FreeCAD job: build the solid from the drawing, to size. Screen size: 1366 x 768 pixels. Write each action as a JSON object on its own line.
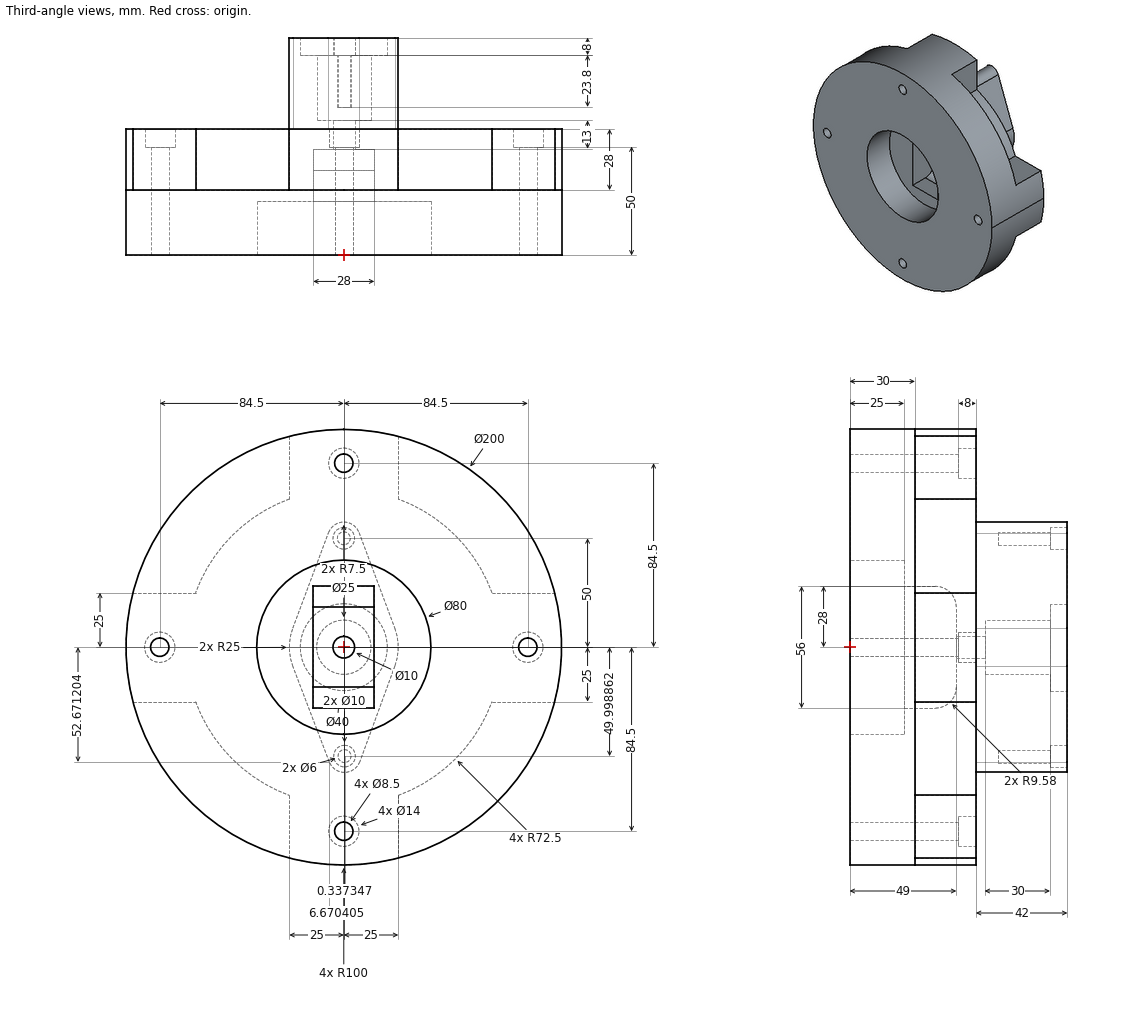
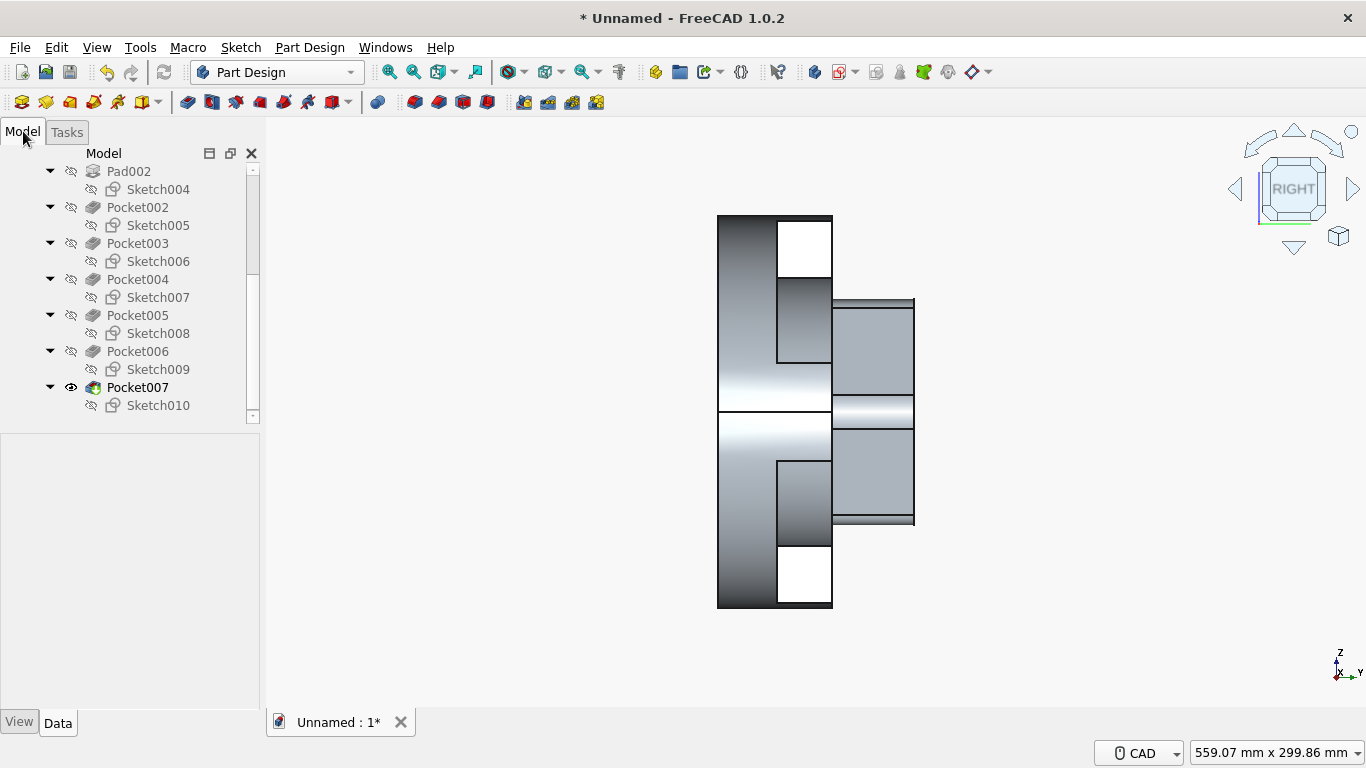
{"action": "scroll", "coordinate": [140, 293], "scroll_direction": "down", "scroll_amount": 3}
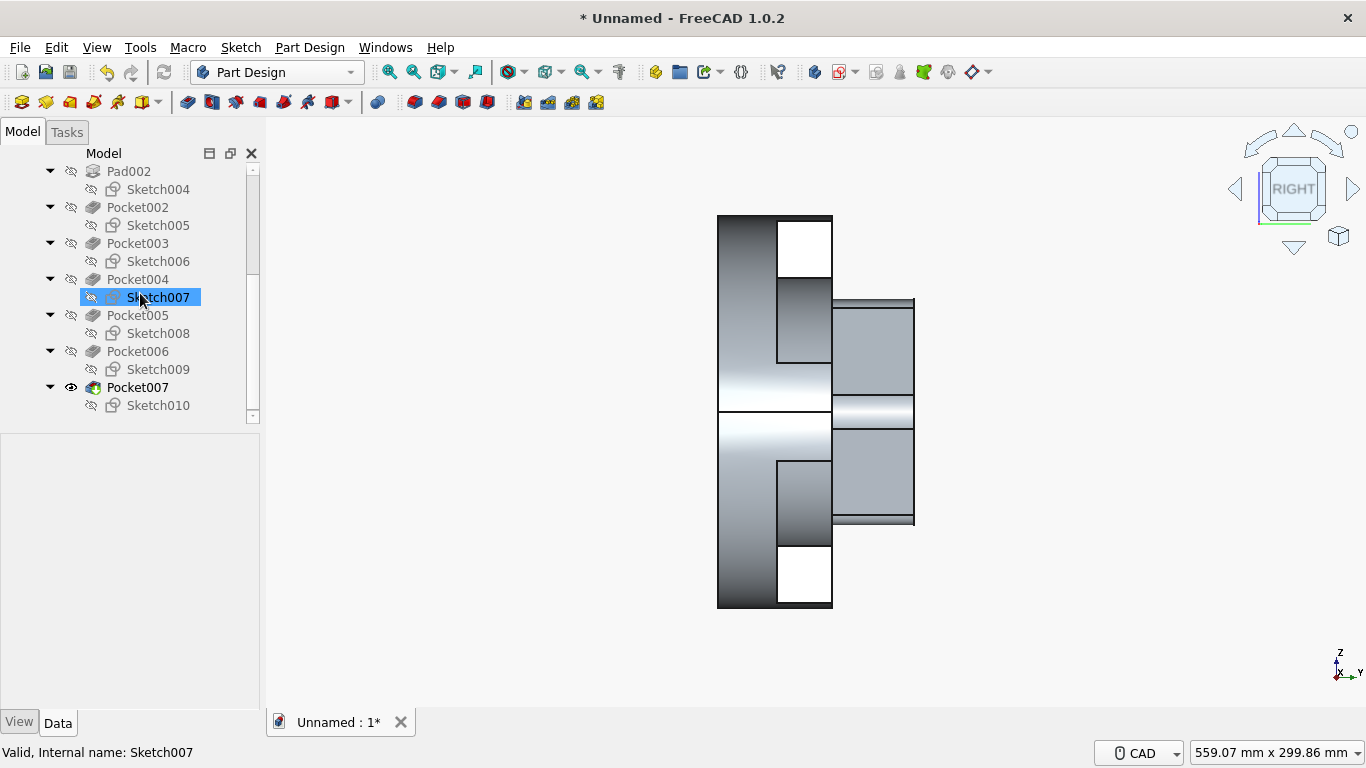
{"action": "scroll", "coordinate": [140, 293], "scroll_direction": "up", "scroll_amount": 15}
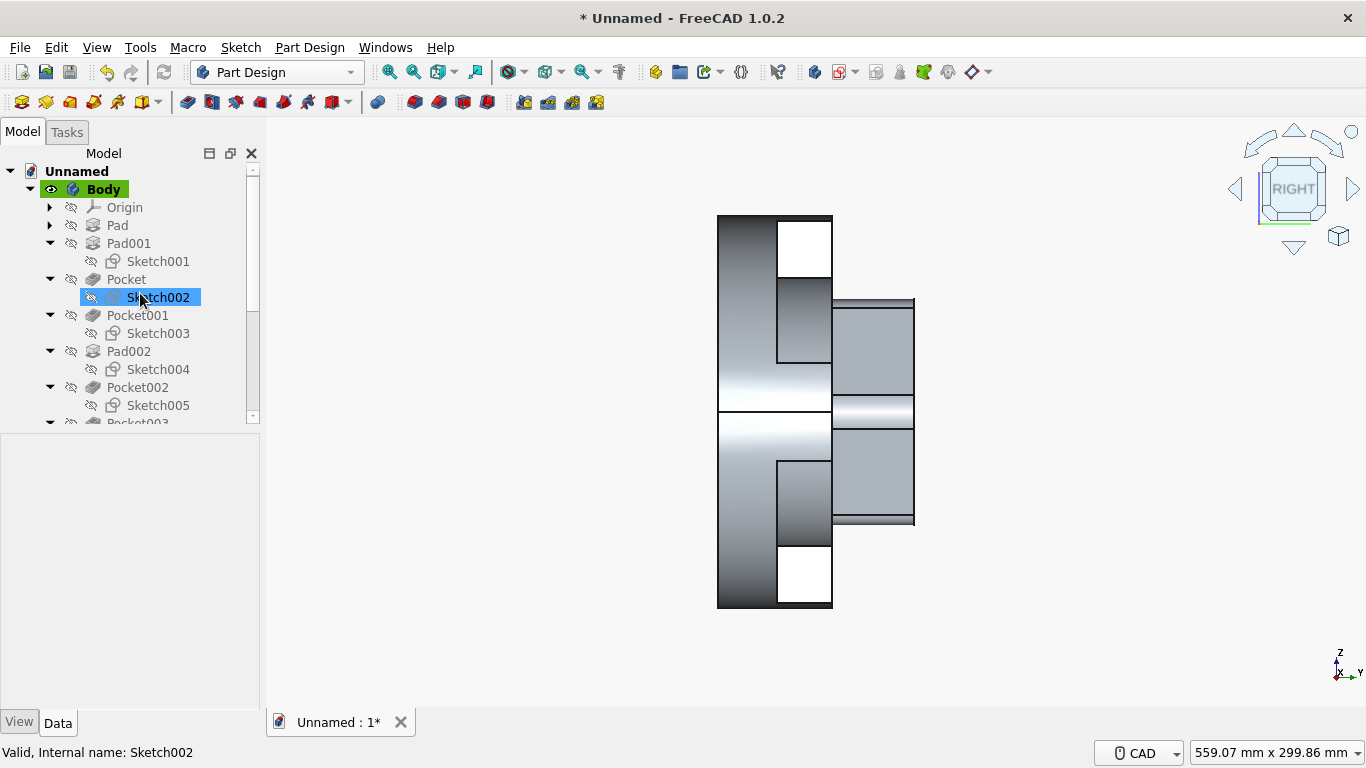
{"action": "left_click", "coordinate": [50, 207]}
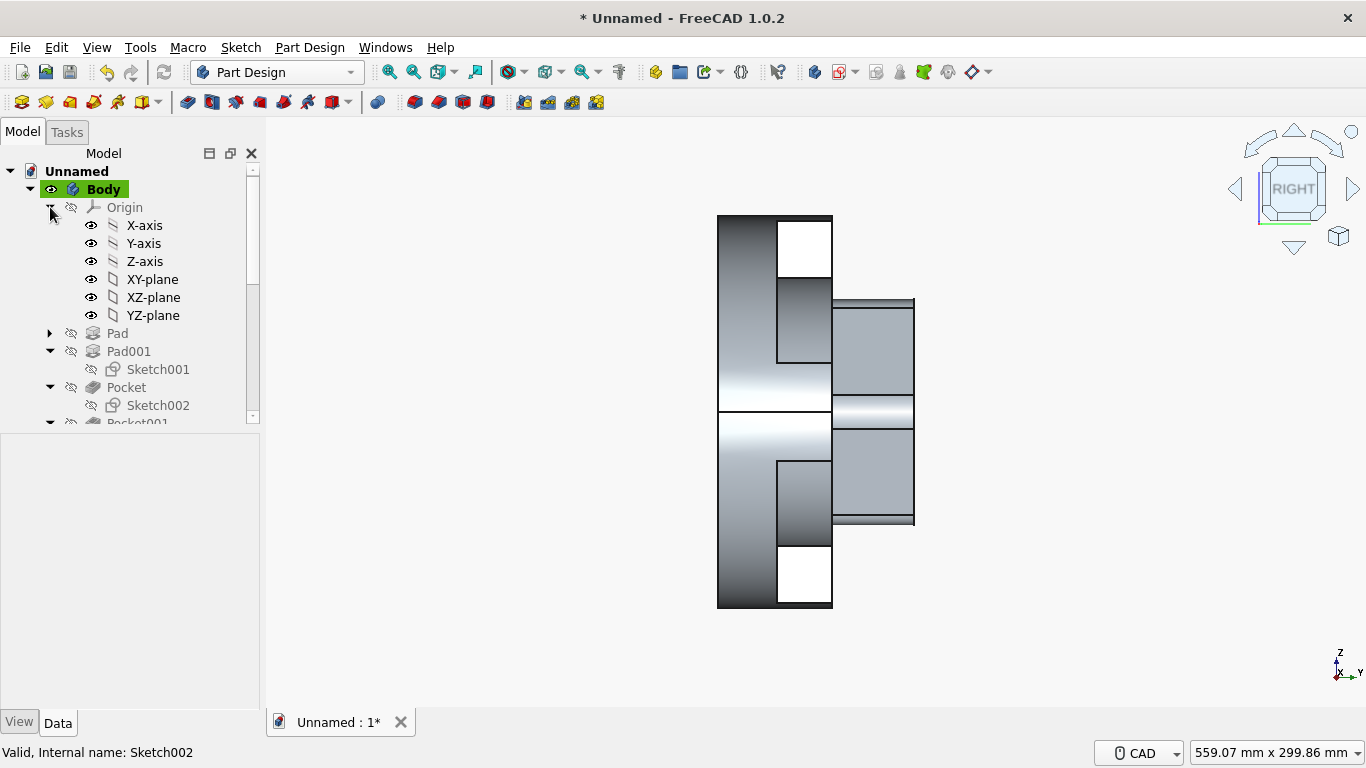
{"action": "left_click", "coordinate": [136, 297]}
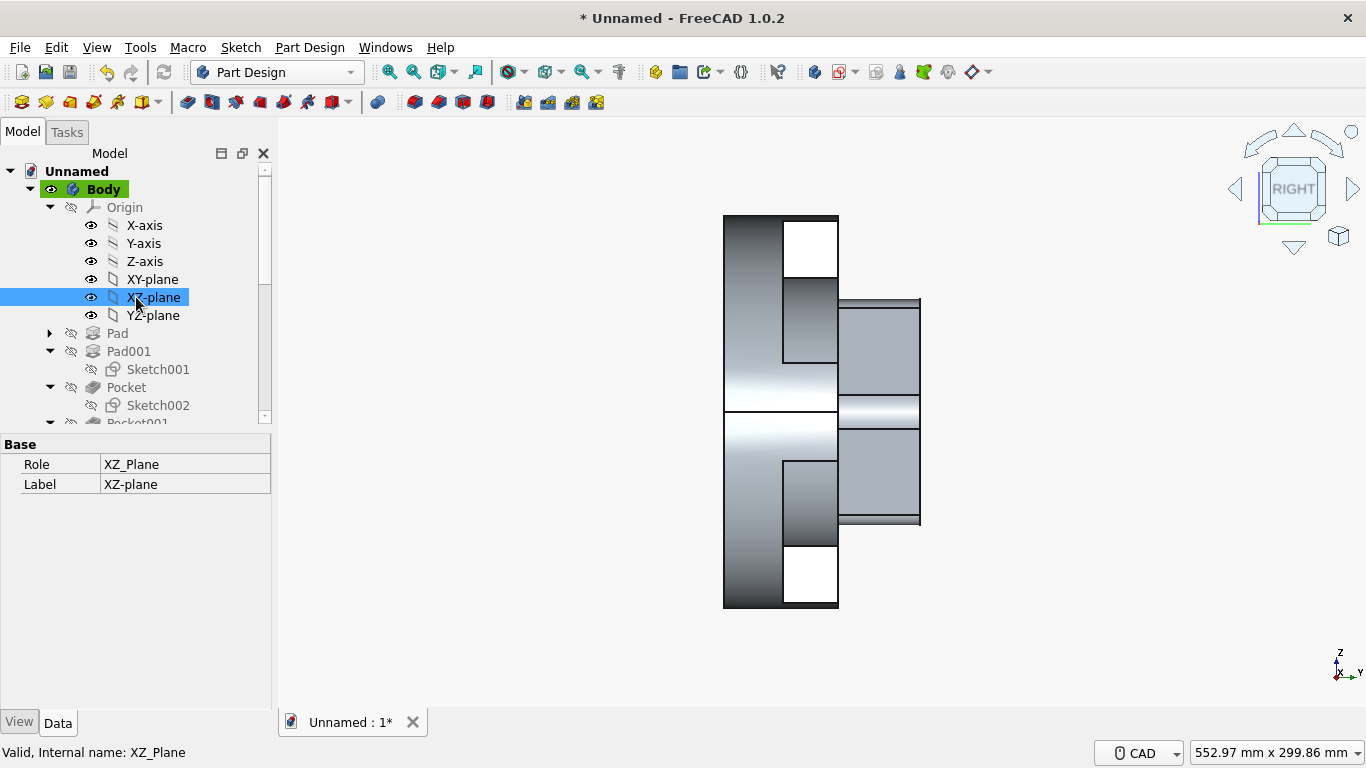
{"action": "left_click", "coordinate": [972, 72]}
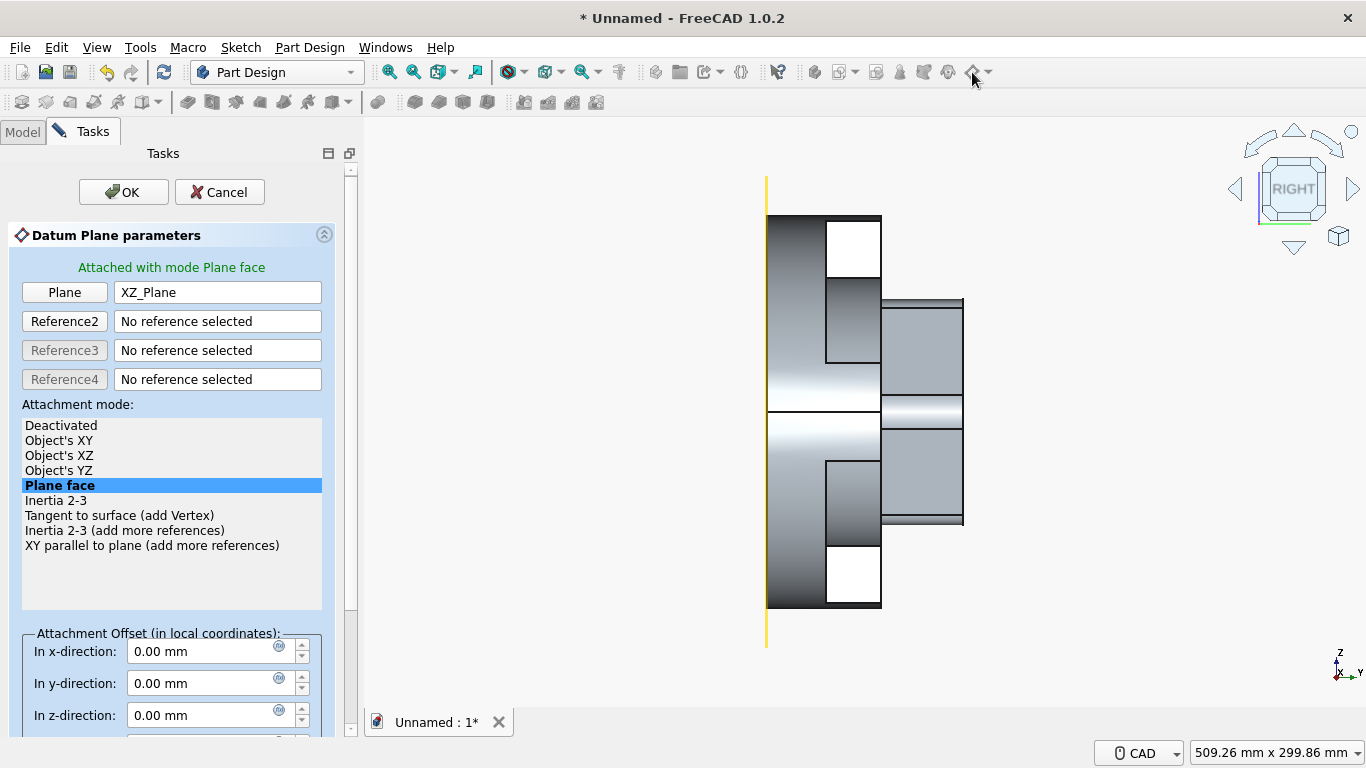
{"action": "triple_click", "coordinate": [210, 715]}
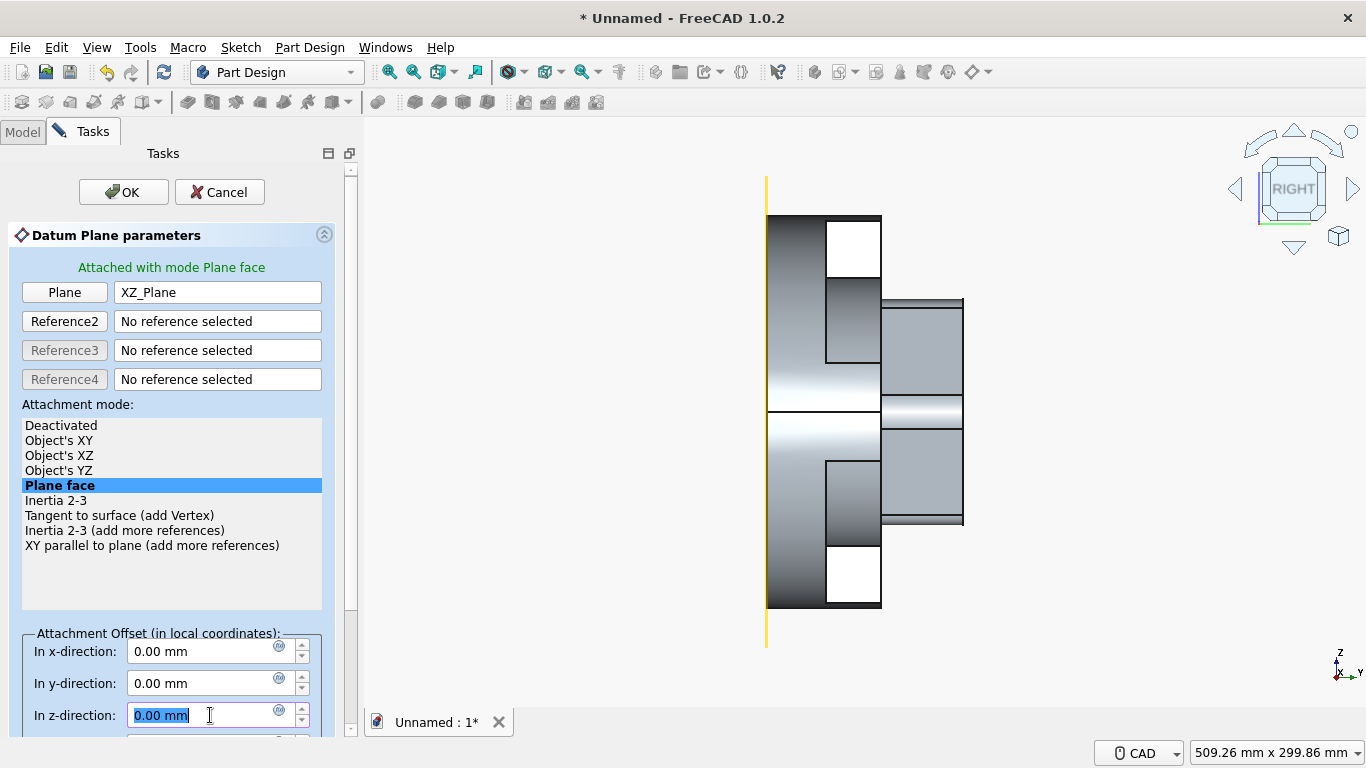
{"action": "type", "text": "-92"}
{"action": "key", "text": "Tab"}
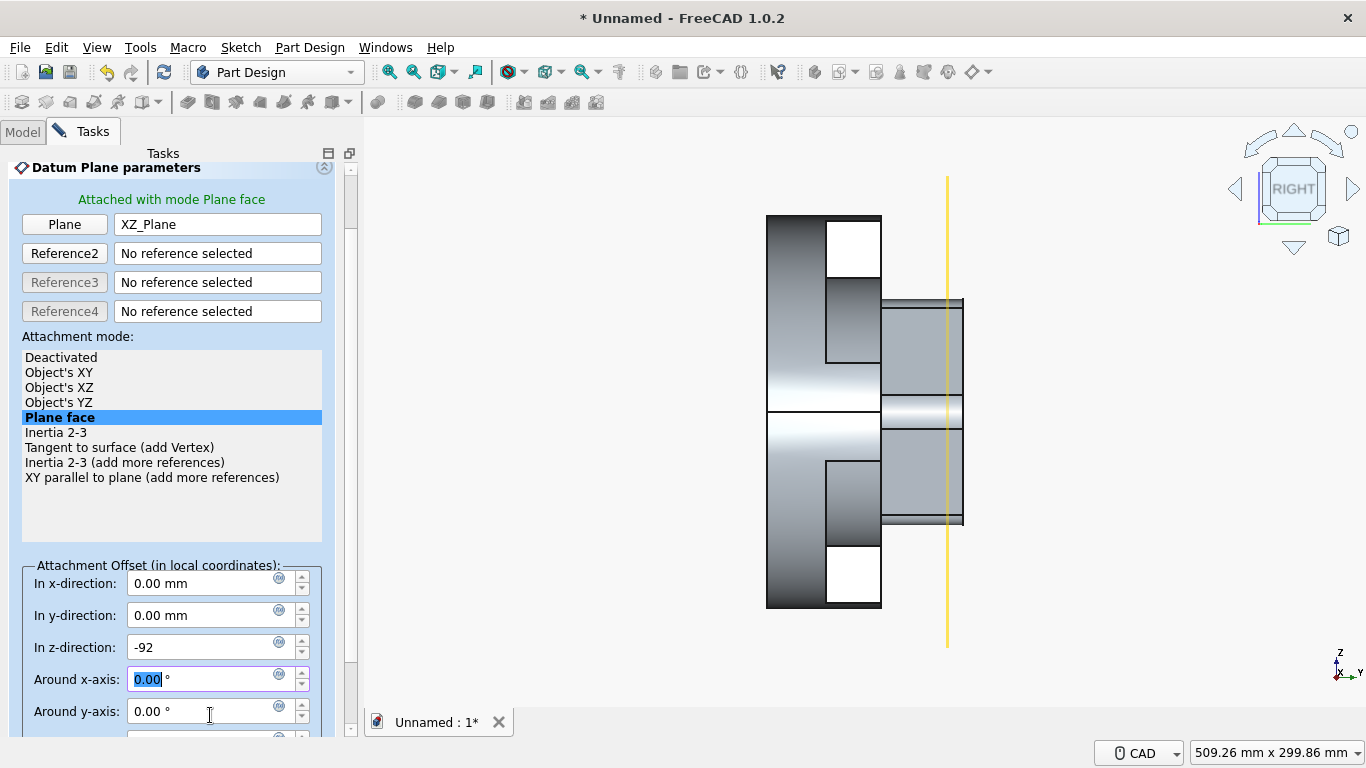
{"action": "scroll", "coordinate": [351, 450], "scroll_direction": "up", "scroll_amount": 2}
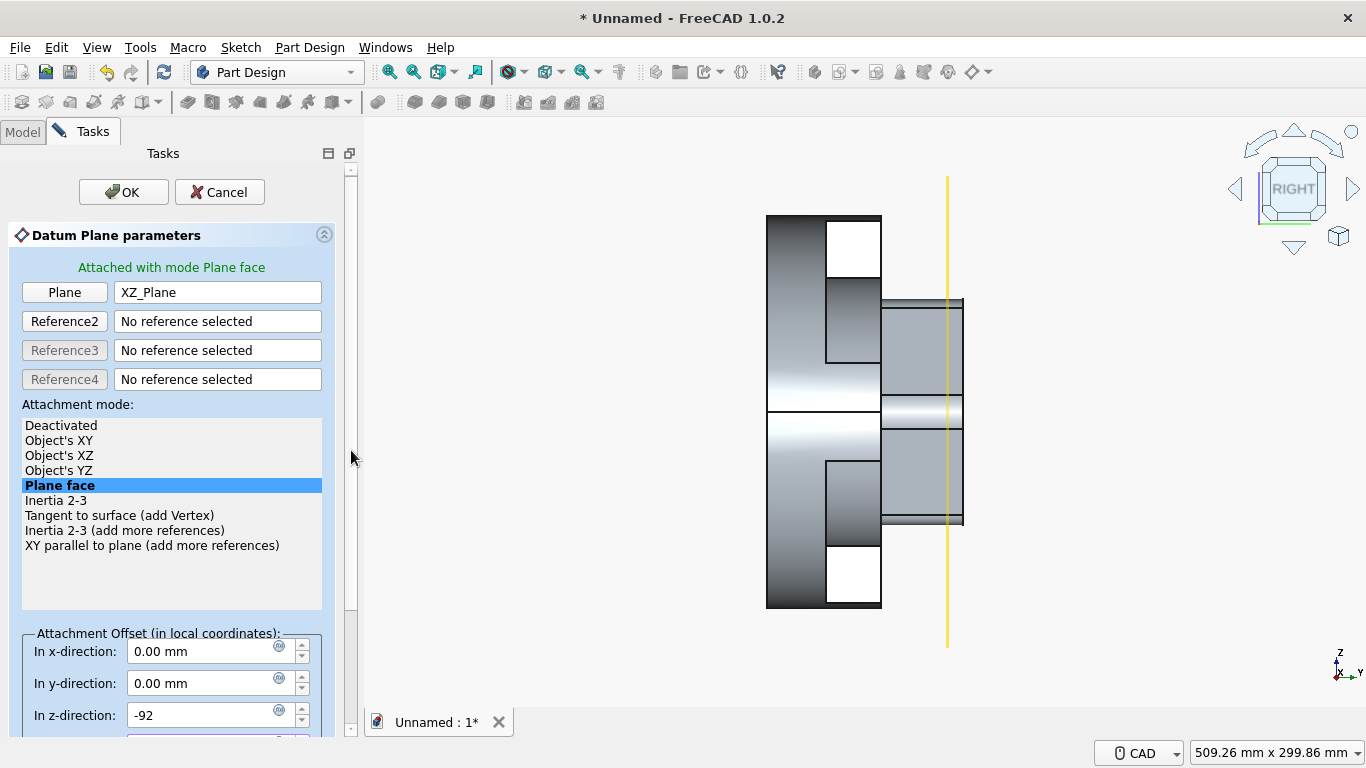
{"action": "left_click", "coordinate": [124, 192]}